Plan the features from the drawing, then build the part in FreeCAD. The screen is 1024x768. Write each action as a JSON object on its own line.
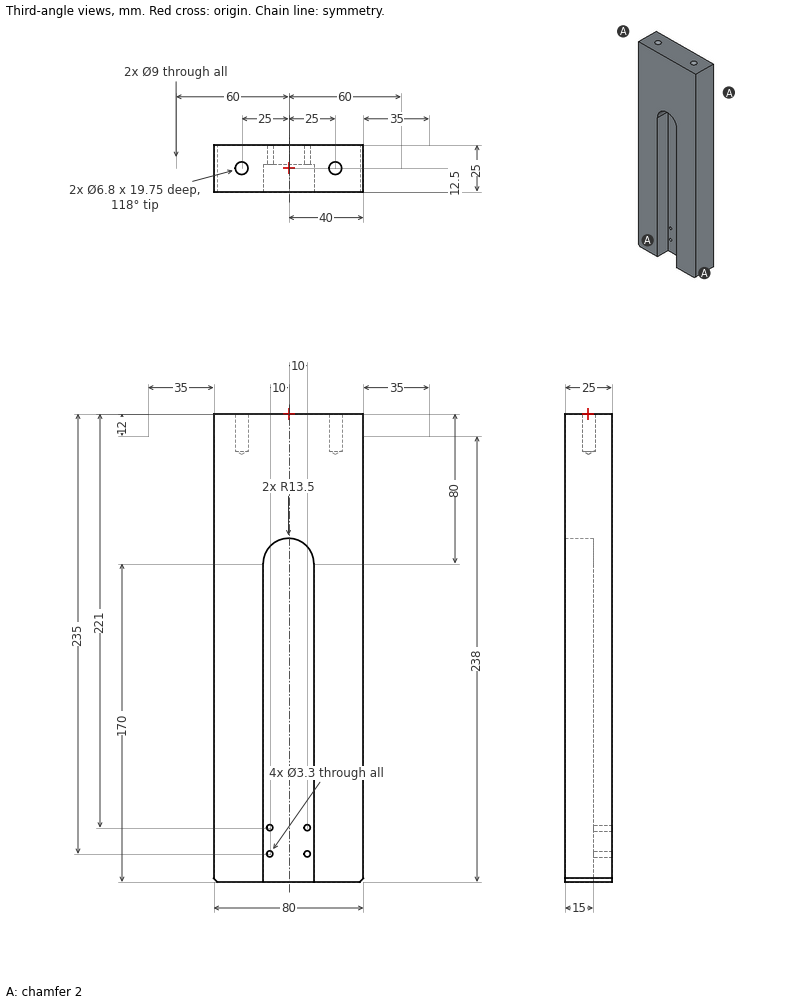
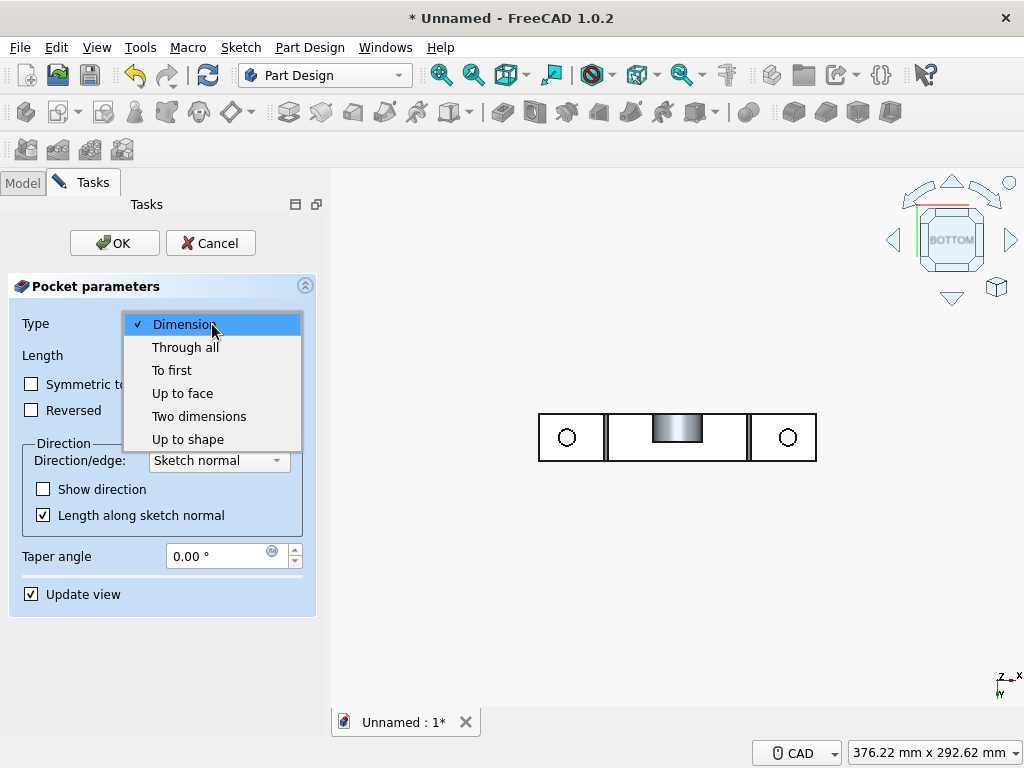
{"action": "left_click", "coordinate": [212, 348]}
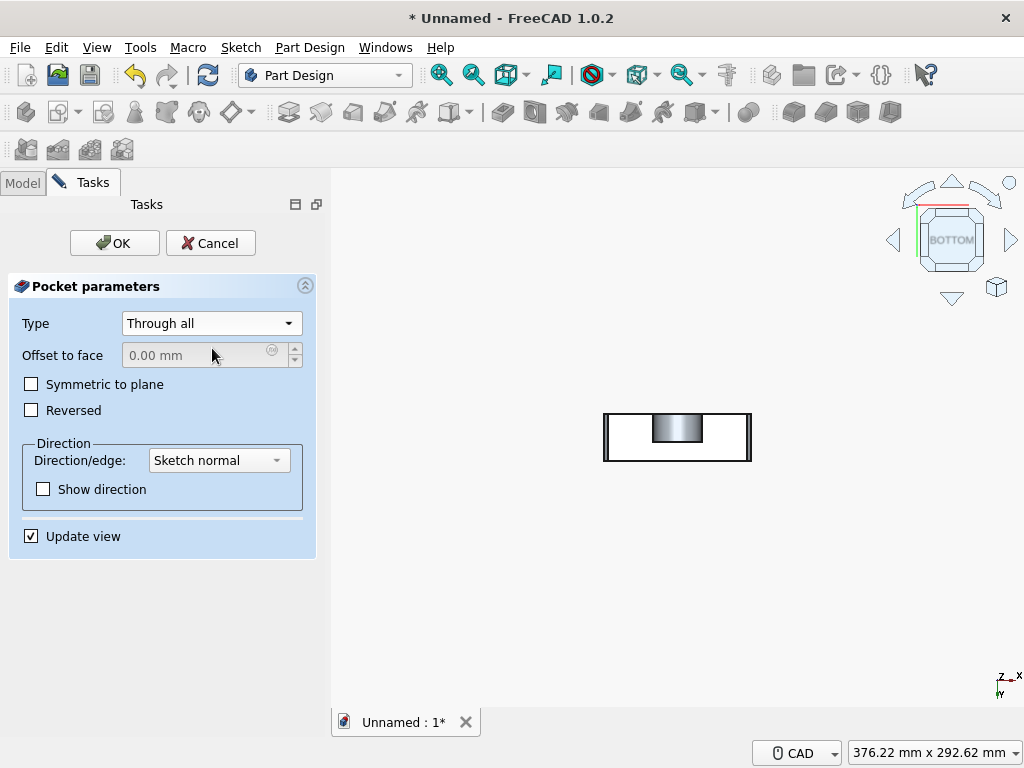
{"action": "left_click", "coordinate": [115, 243]}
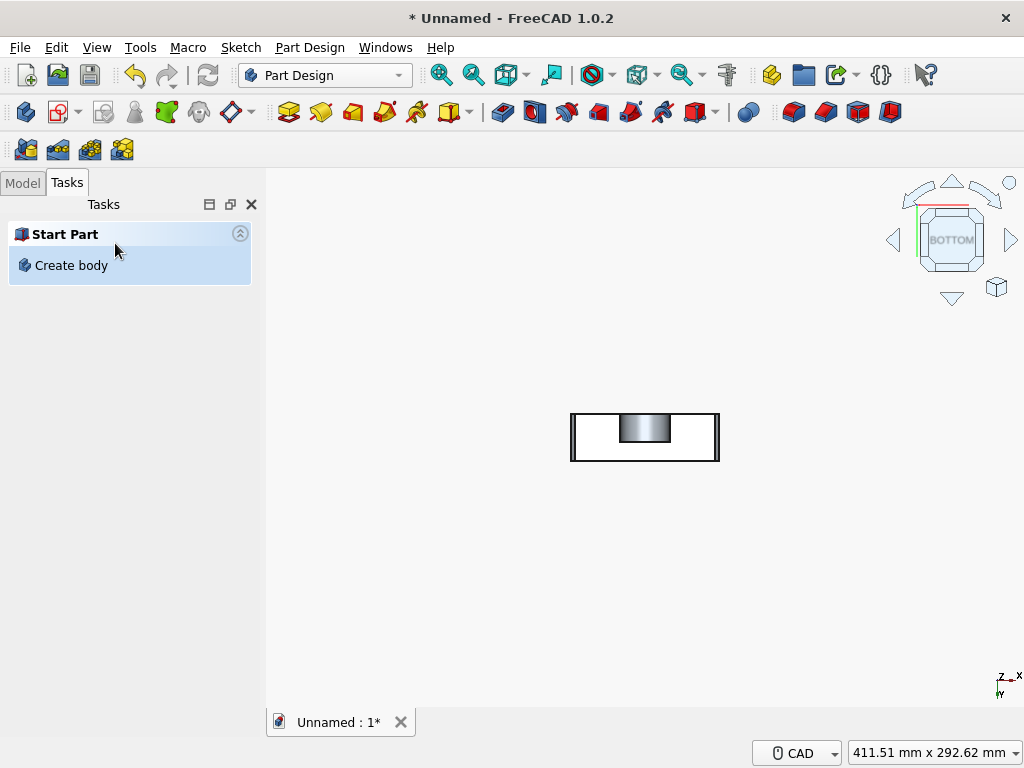
{"action": "left_click", "coordinate": [442, 76]}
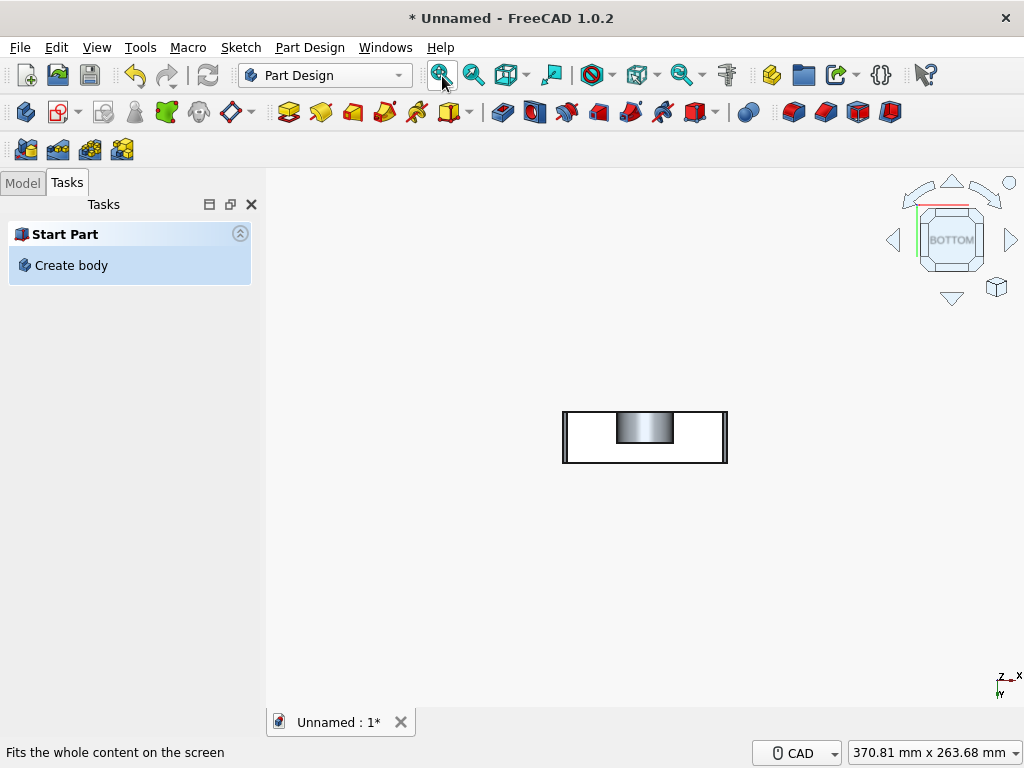
{"action": "left_click", "coordinate": [58, 112]}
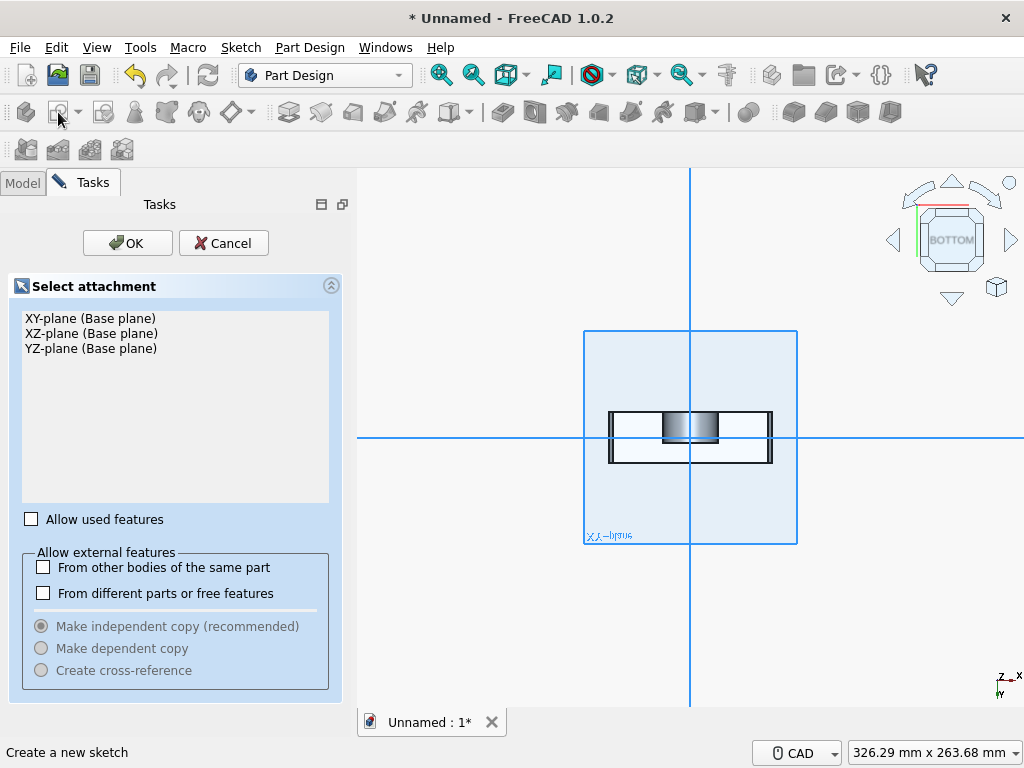
{"action": "left_click", "coordinate": [82, 318]}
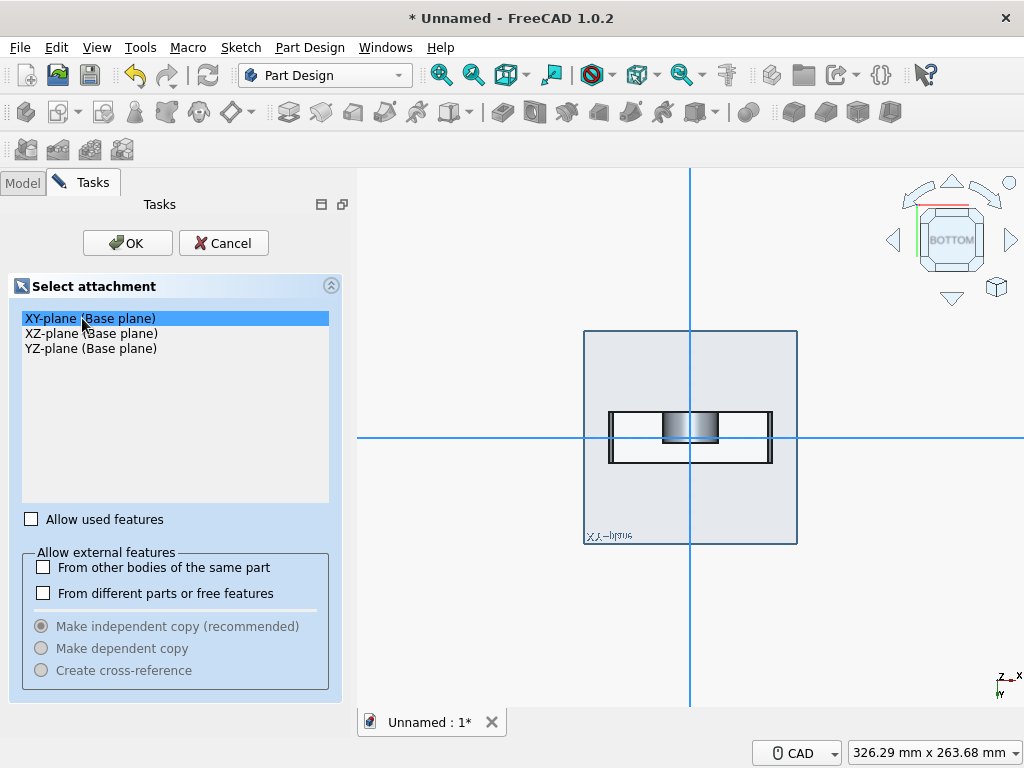
{"action": "left_click", "coordinate": [128, 243]}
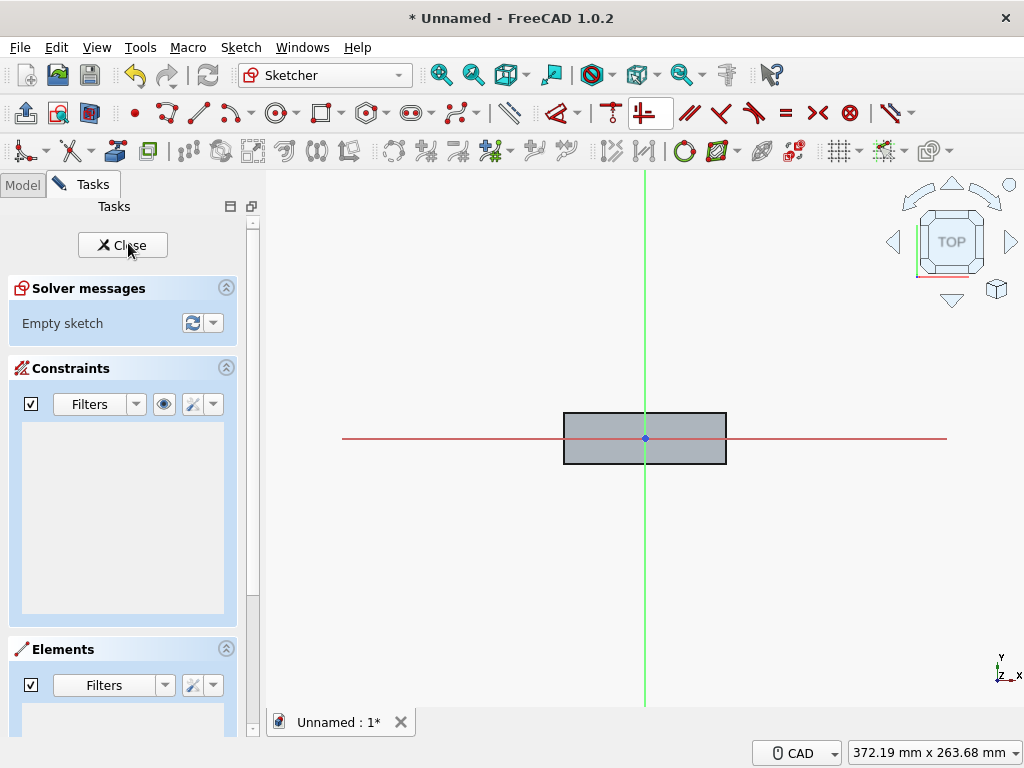
{"action": "scroll", "coordinate": [675, 439], "scroll_direction": "up", "scroll_amount": 6}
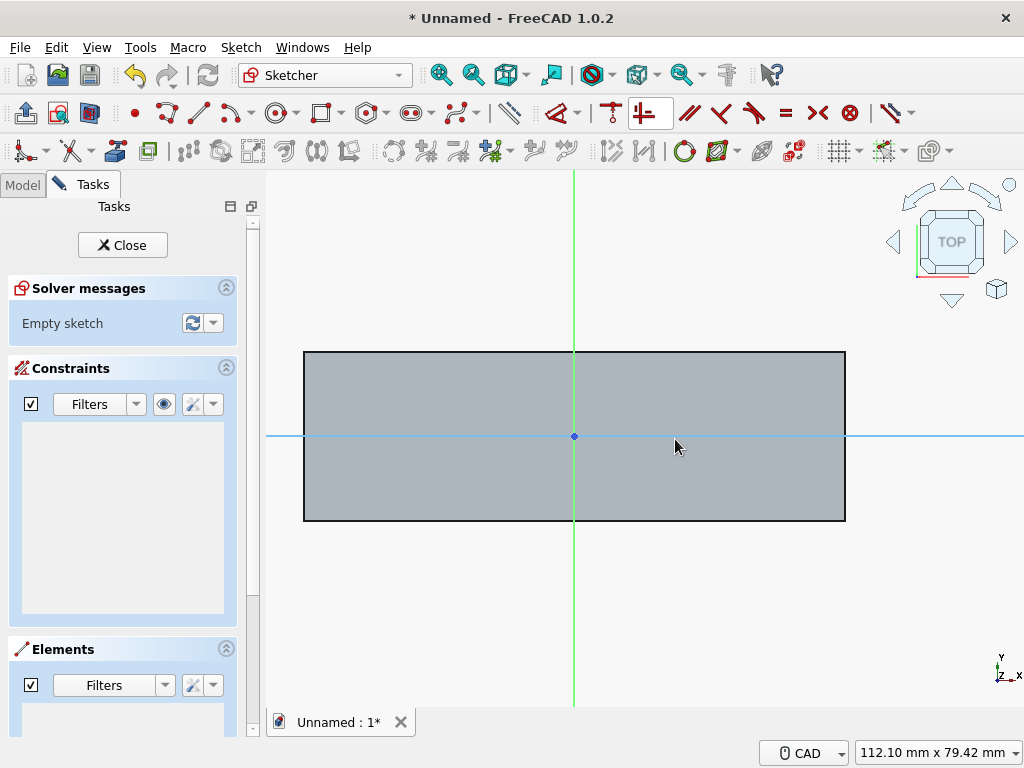
{"action": "left_click", "coordinate": [276, 114]}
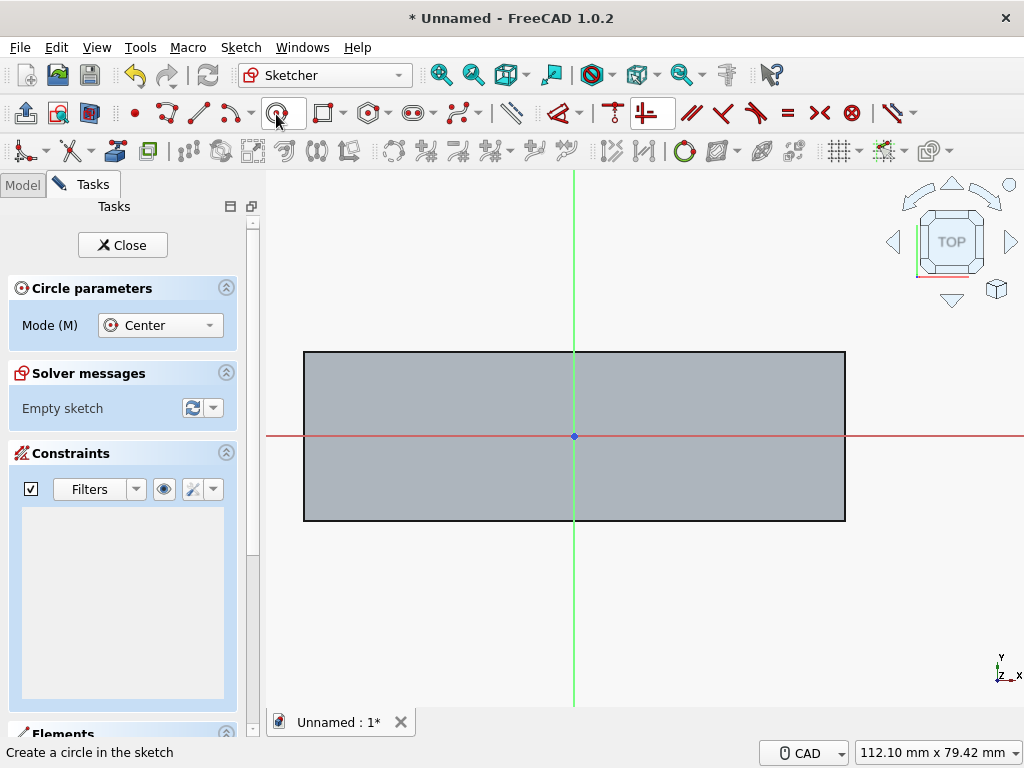
{"action": "left_click", "coordinate": [405, 436]}
{"action": "left_click", "coordinate": [421, 420]}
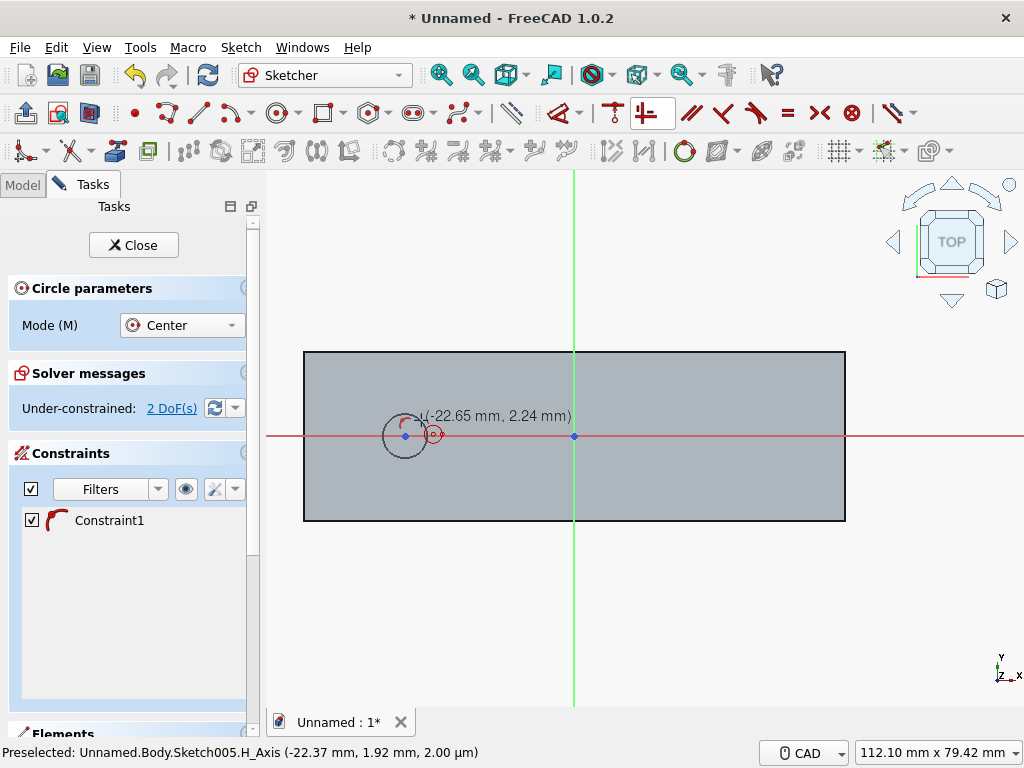
{"action": "left_click", "coordinate": [743, 436]}
{"action": "left_click", "coordinate": [759, 420]}
{"action": "key", "text": "Escape"}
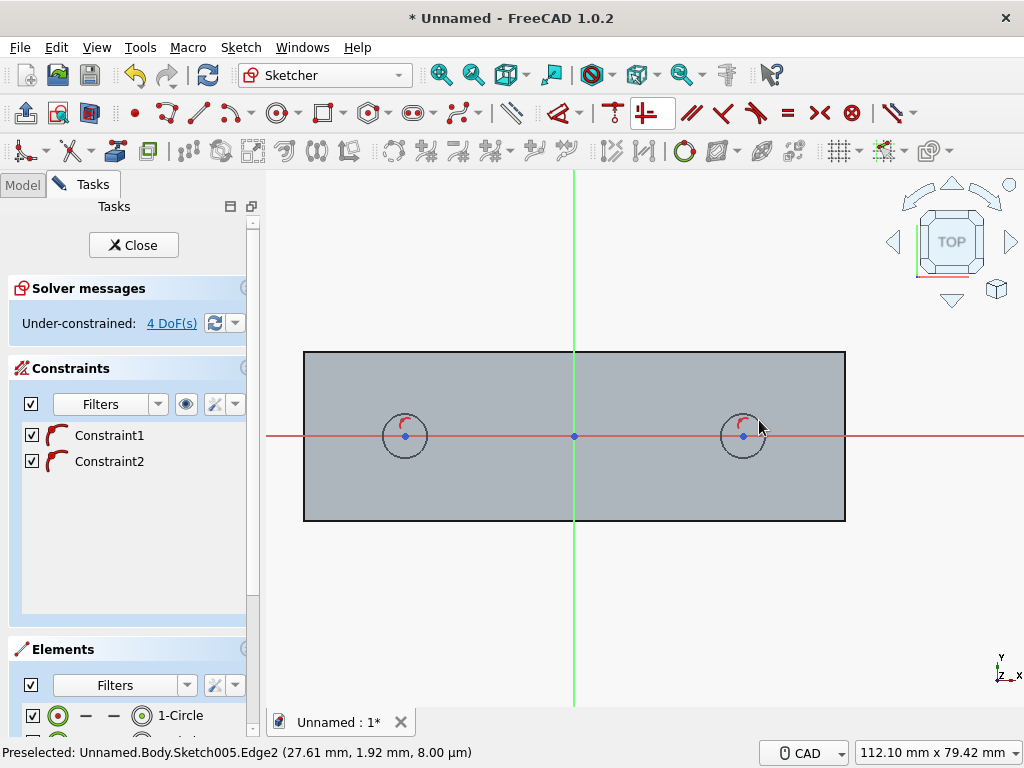
{"action": "left_click", "coordinate": [421, 421]}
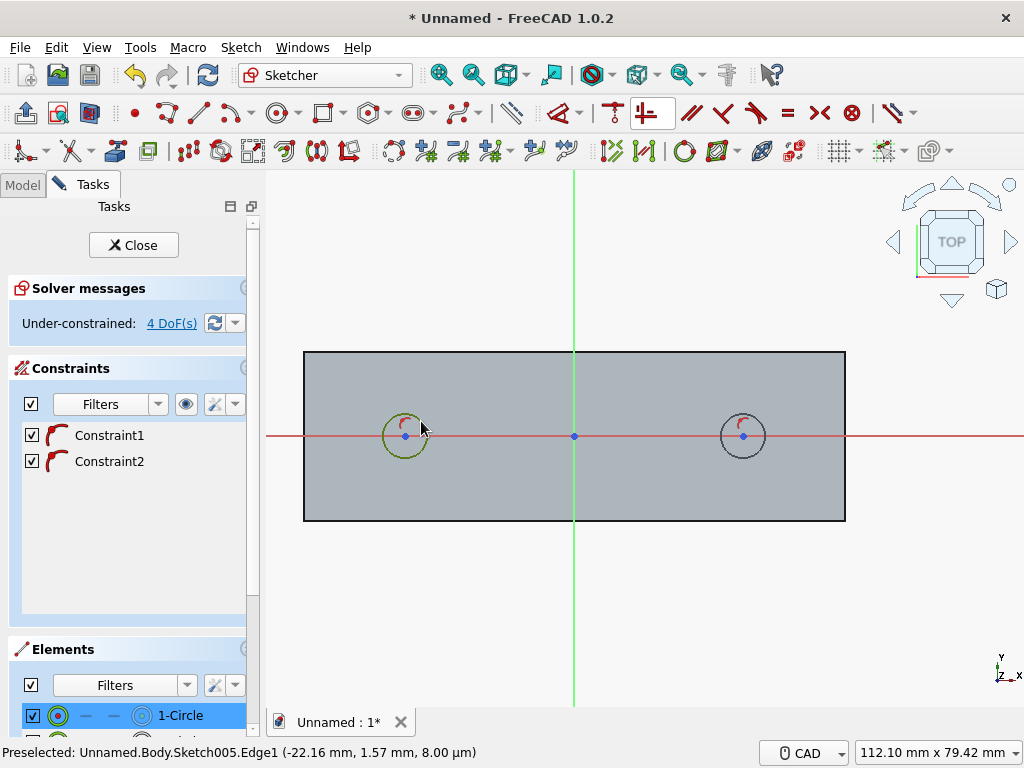
{"action": "left_click", "coordinate": [759, 421]}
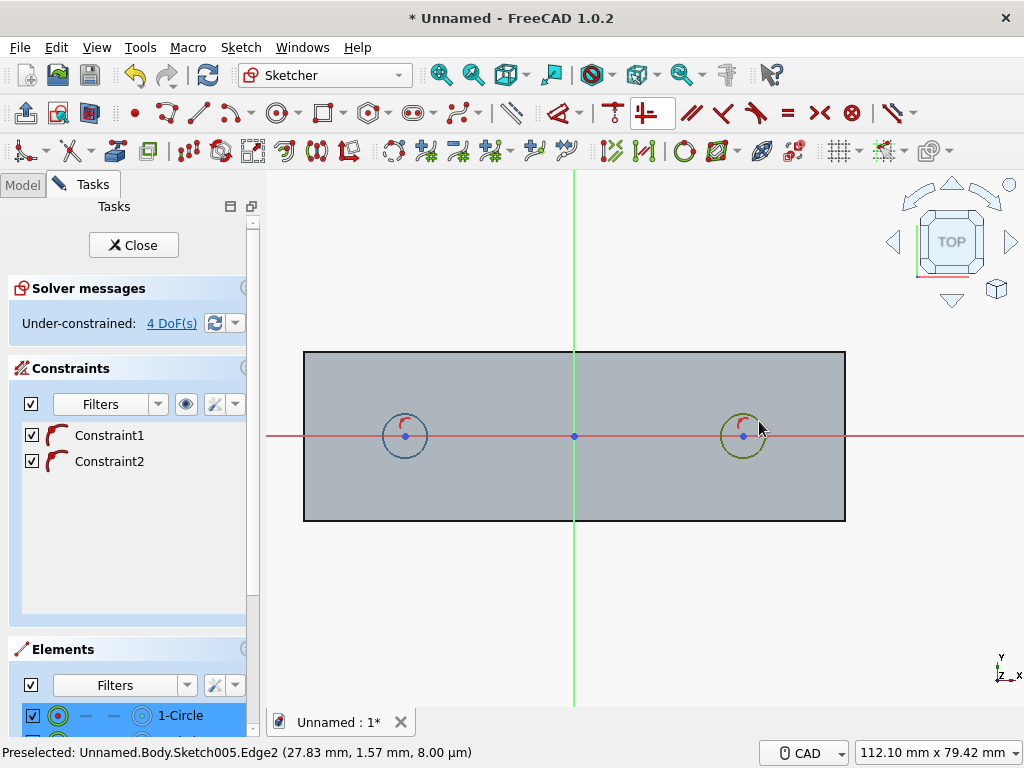
{"action": "left_click", "coordinate": [788, 114]}